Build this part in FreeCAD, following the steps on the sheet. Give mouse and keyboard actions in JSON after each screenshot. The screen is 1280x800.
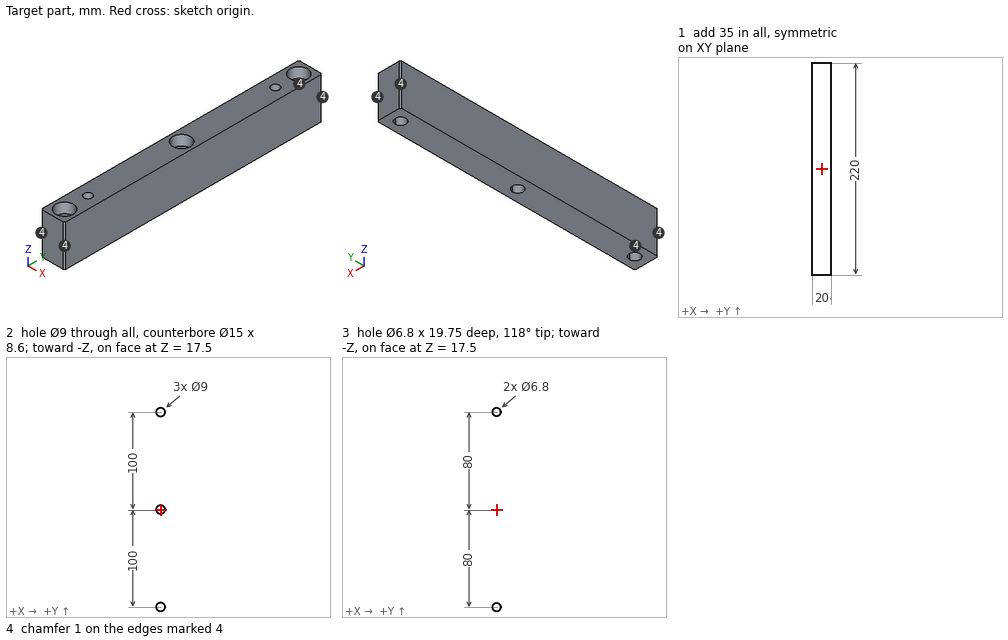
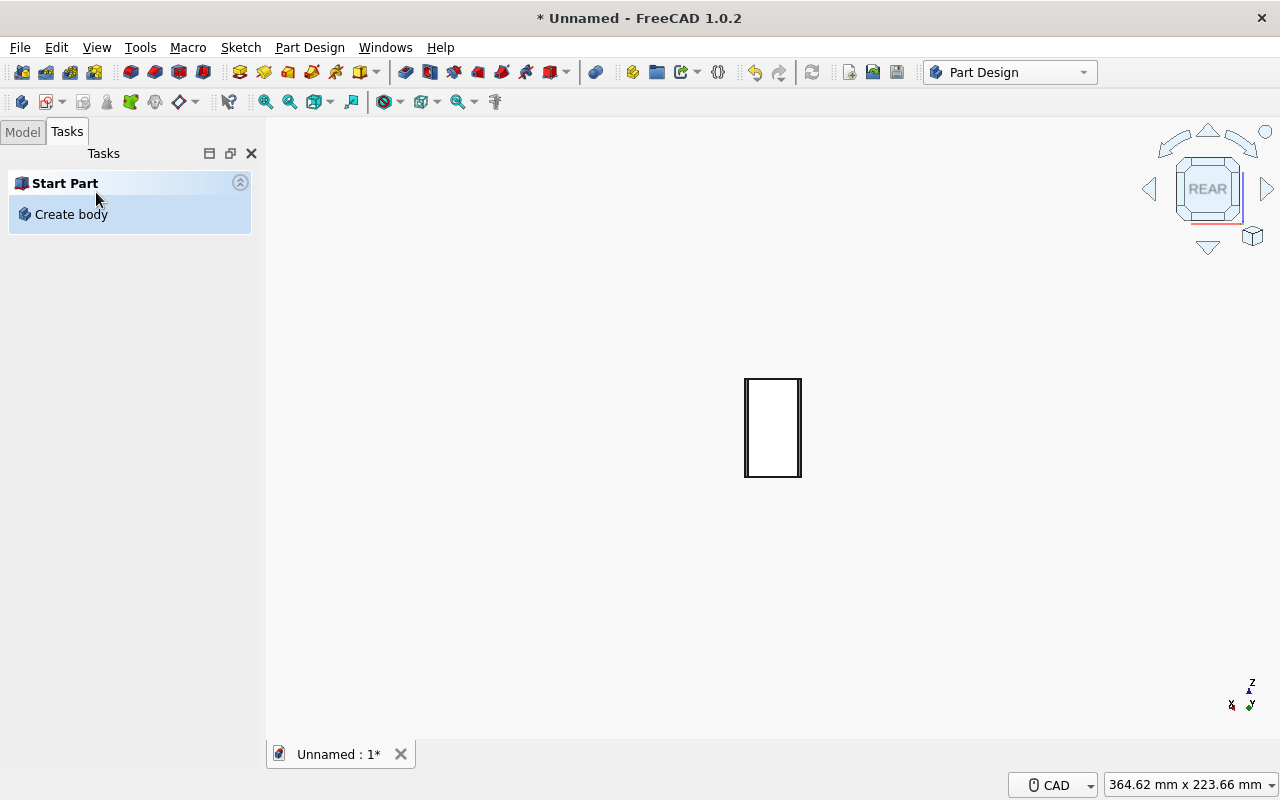
{"action": "key", "text": "0"}